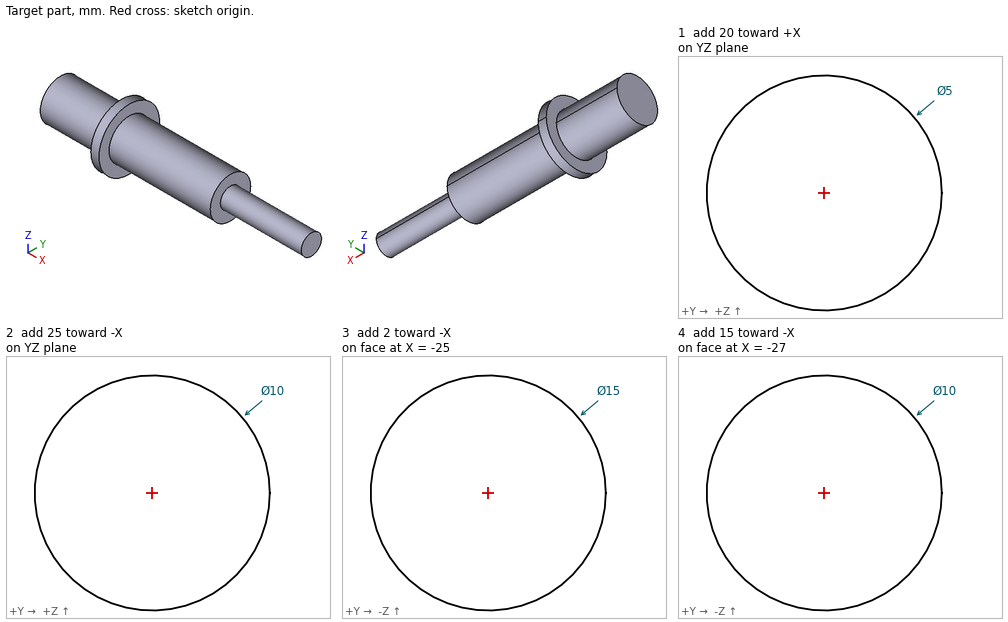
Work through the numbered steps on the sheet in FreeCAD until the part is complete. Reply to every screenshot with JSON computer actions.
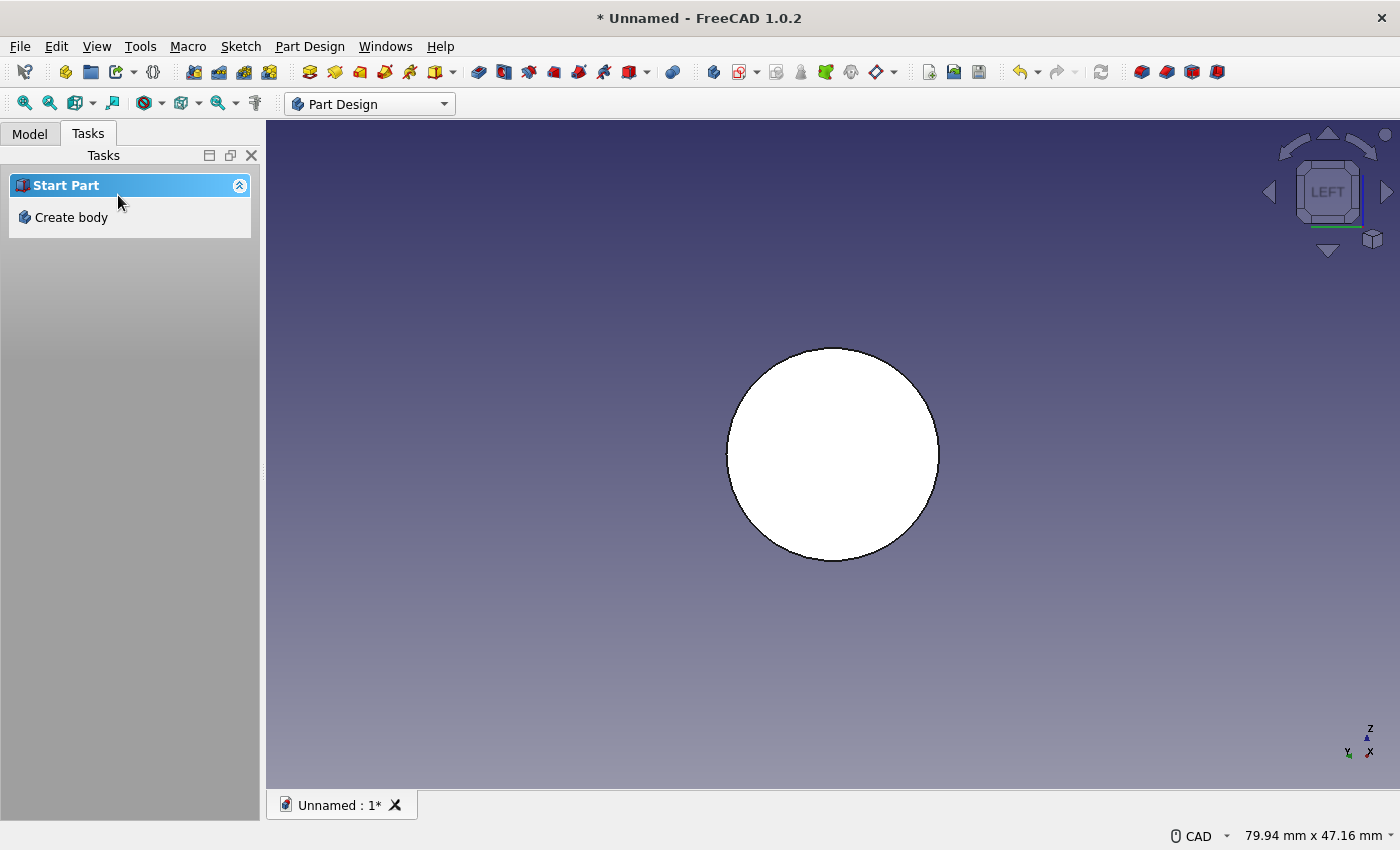
{"action": "key", "text": "v f"}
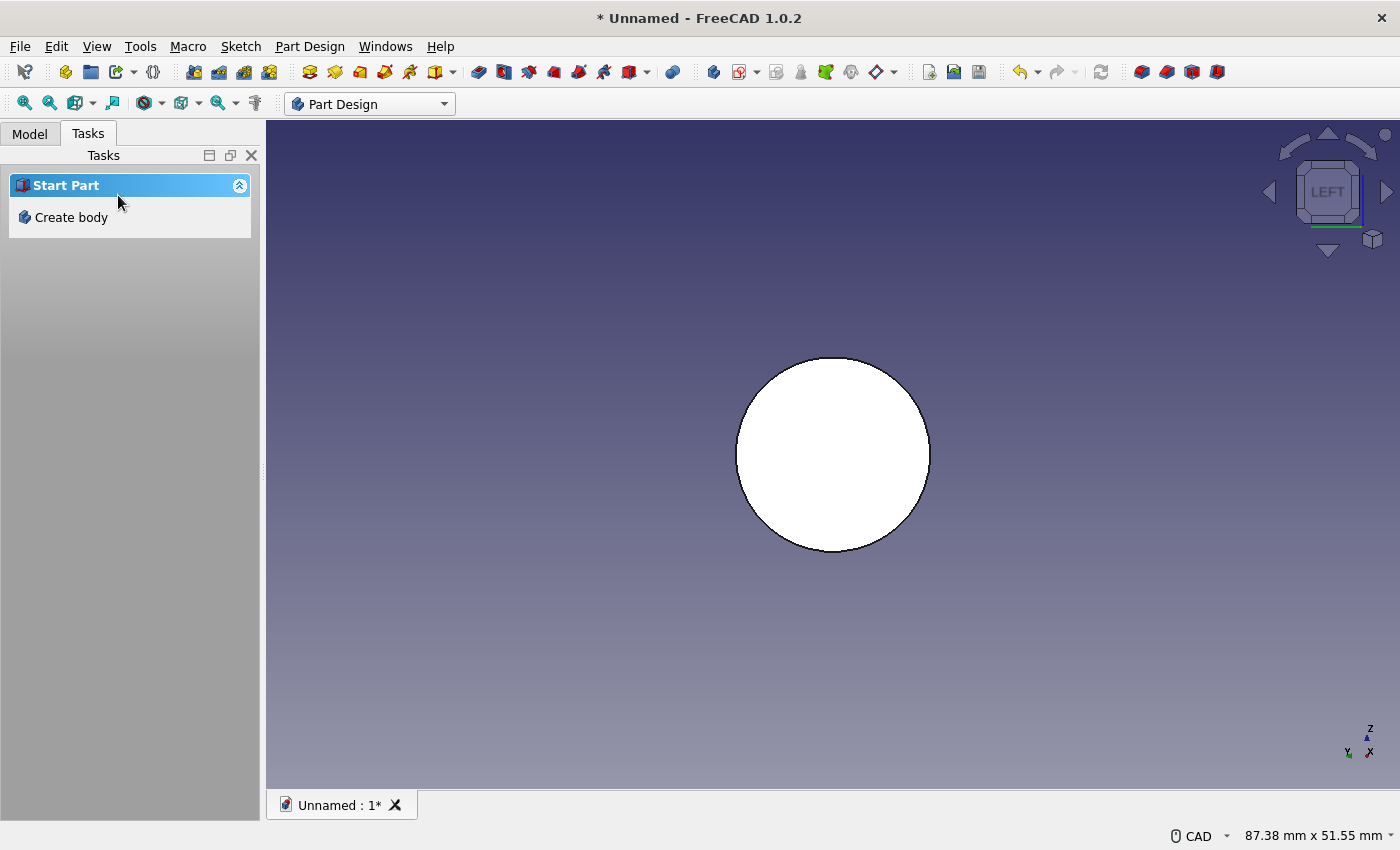
{"action": "left_click", "coordinate": [833, 453]}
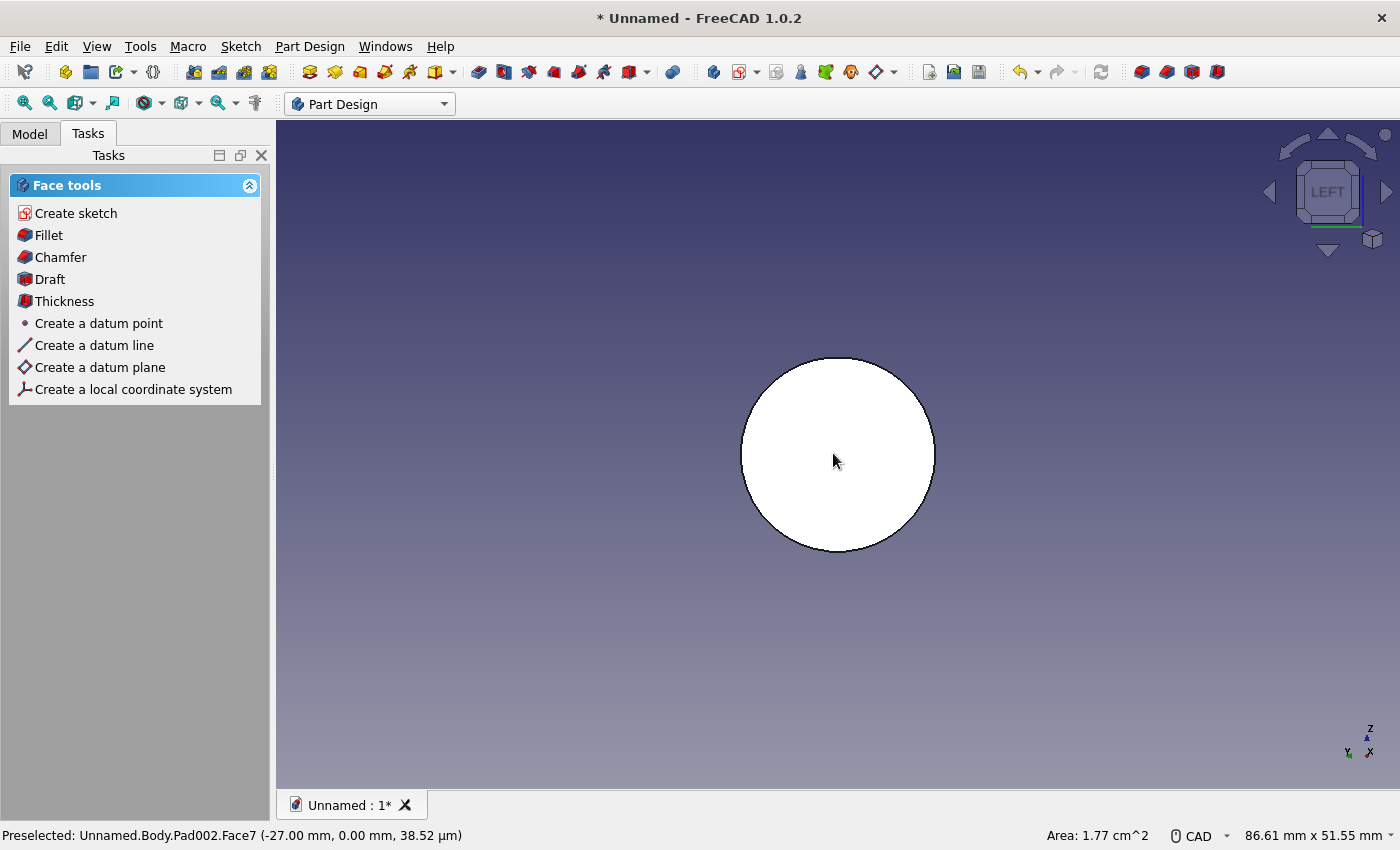
{"action": "left_click", "coordinate": [738, 72]}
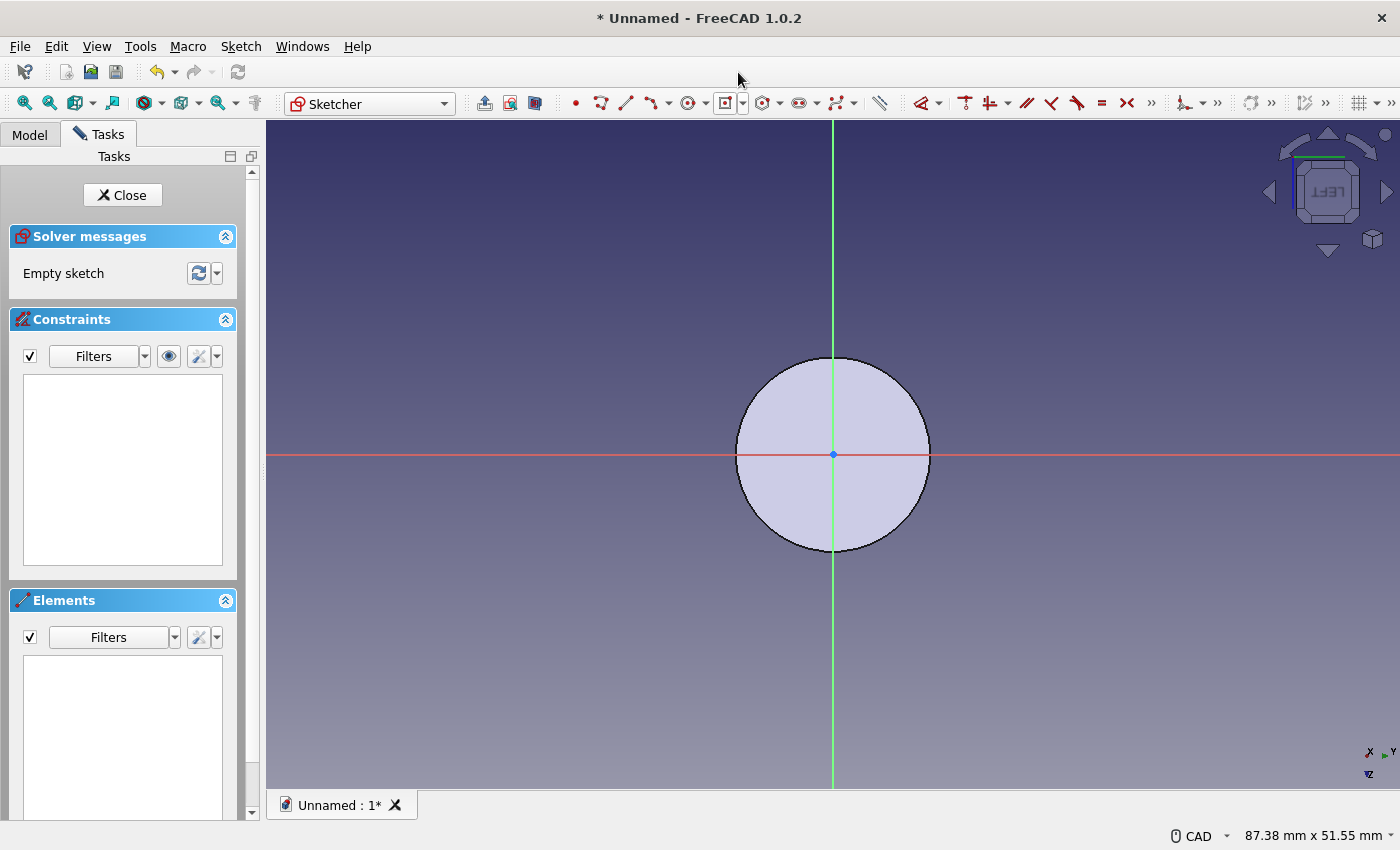
{"action": "scroll", "coordinate": [863, 454], "scroll_direction": "up", "scroll_amount": 6}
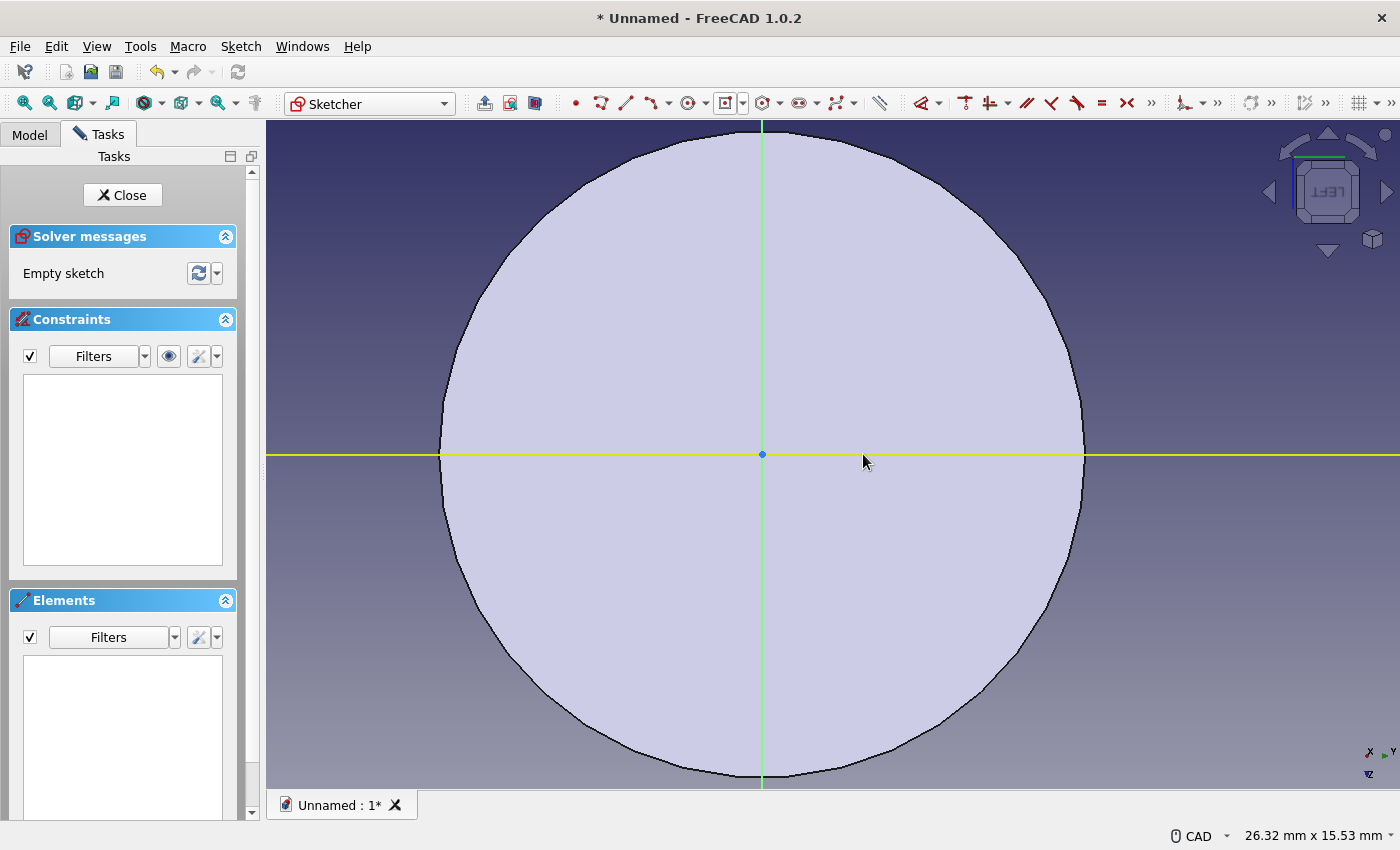
{"action": "key", "text": "g c"}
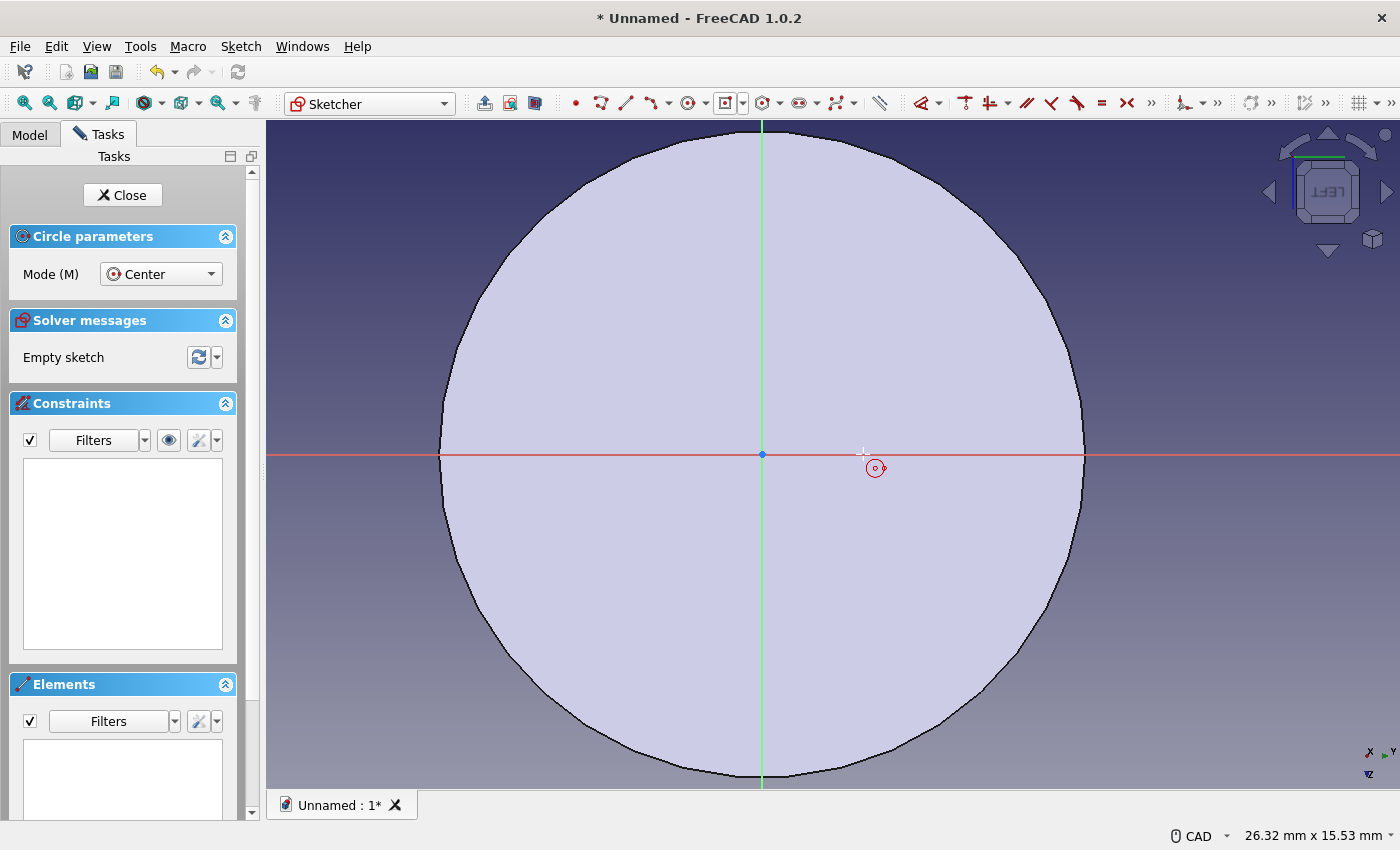
{"action": "left_click", "coordinate": [762, 454]}
{"action": "left_click", "coordinate": [915, 302]}
{"action": "key", "text": "Escape"}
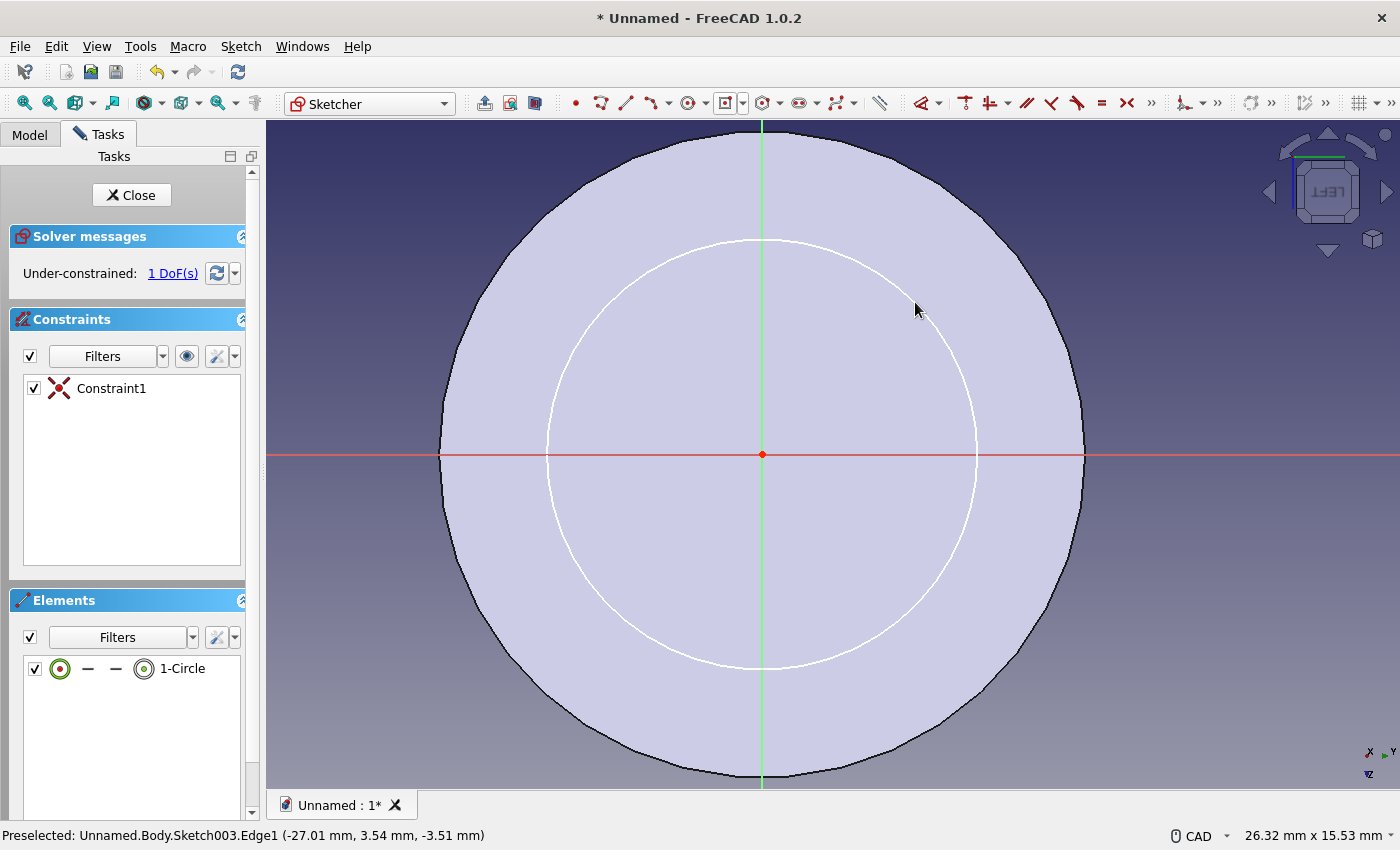
{"action": "key", "text": "d"}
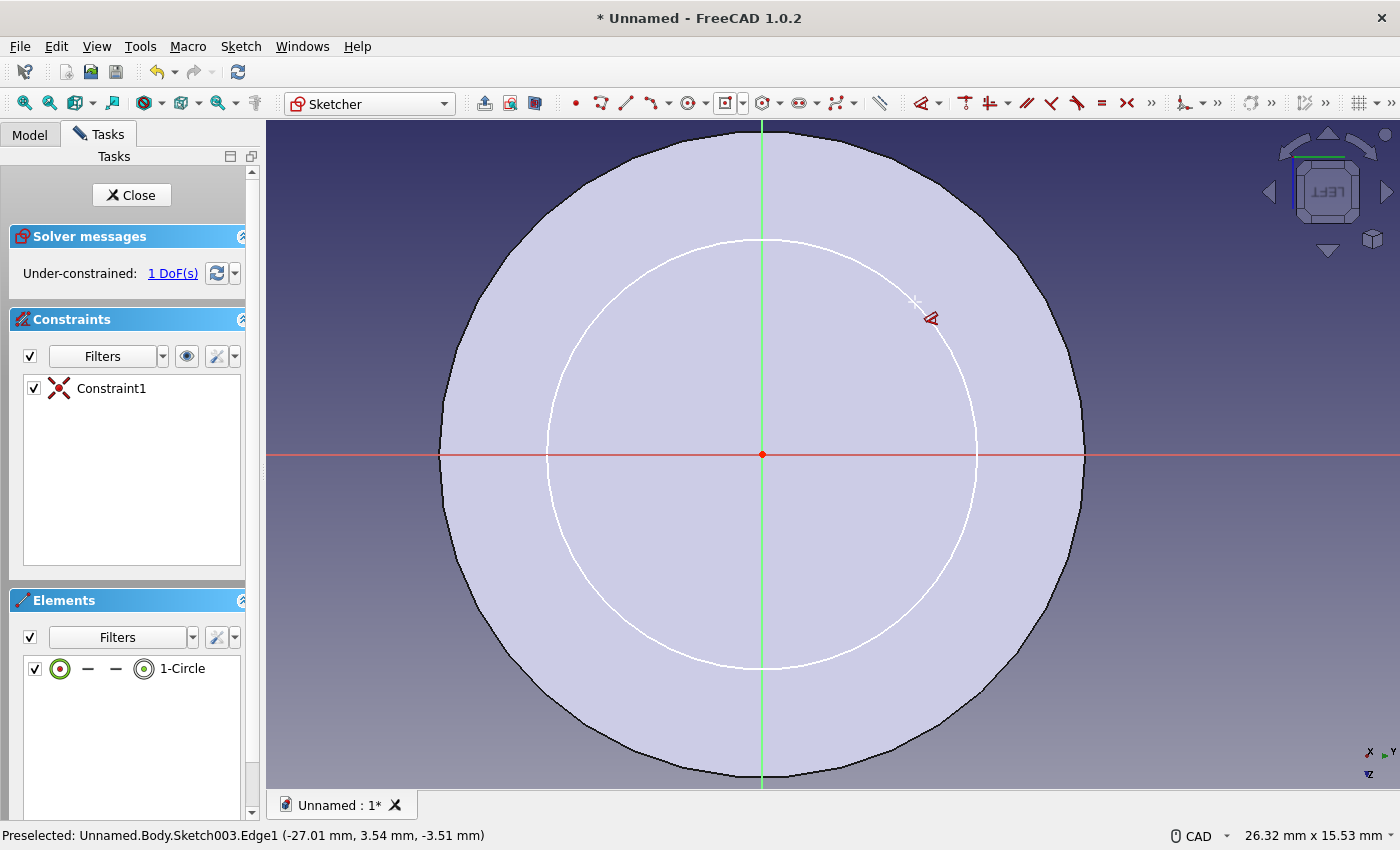
{"action": "left_click", "coordinate": [914, 302]}
{"action": "left_click", "coordinate": [937, 279]}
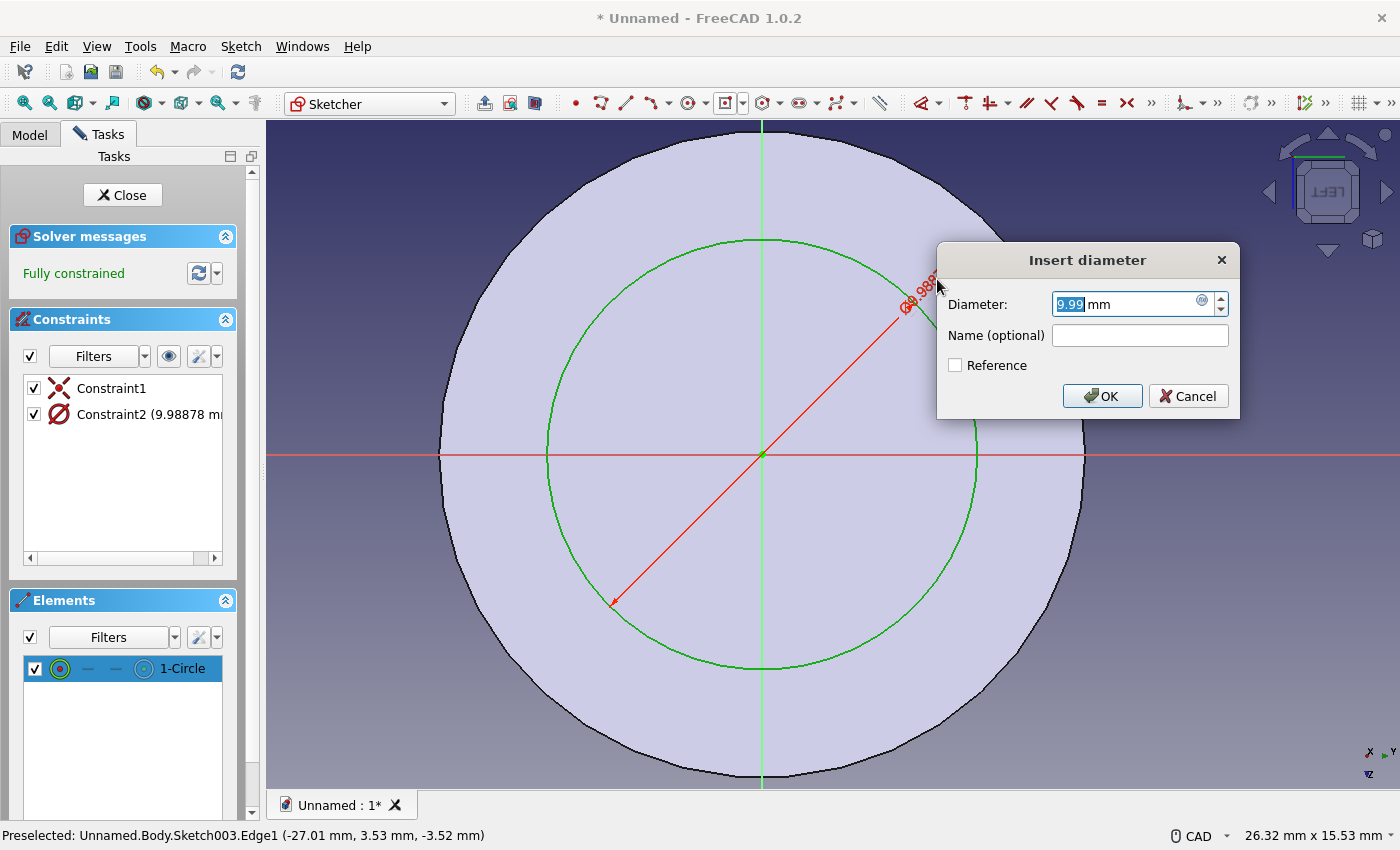
{"action": "type", "text": "10"}
{"action": "key", "text": "Return"}
{"action": "key", "text": "Escape"}